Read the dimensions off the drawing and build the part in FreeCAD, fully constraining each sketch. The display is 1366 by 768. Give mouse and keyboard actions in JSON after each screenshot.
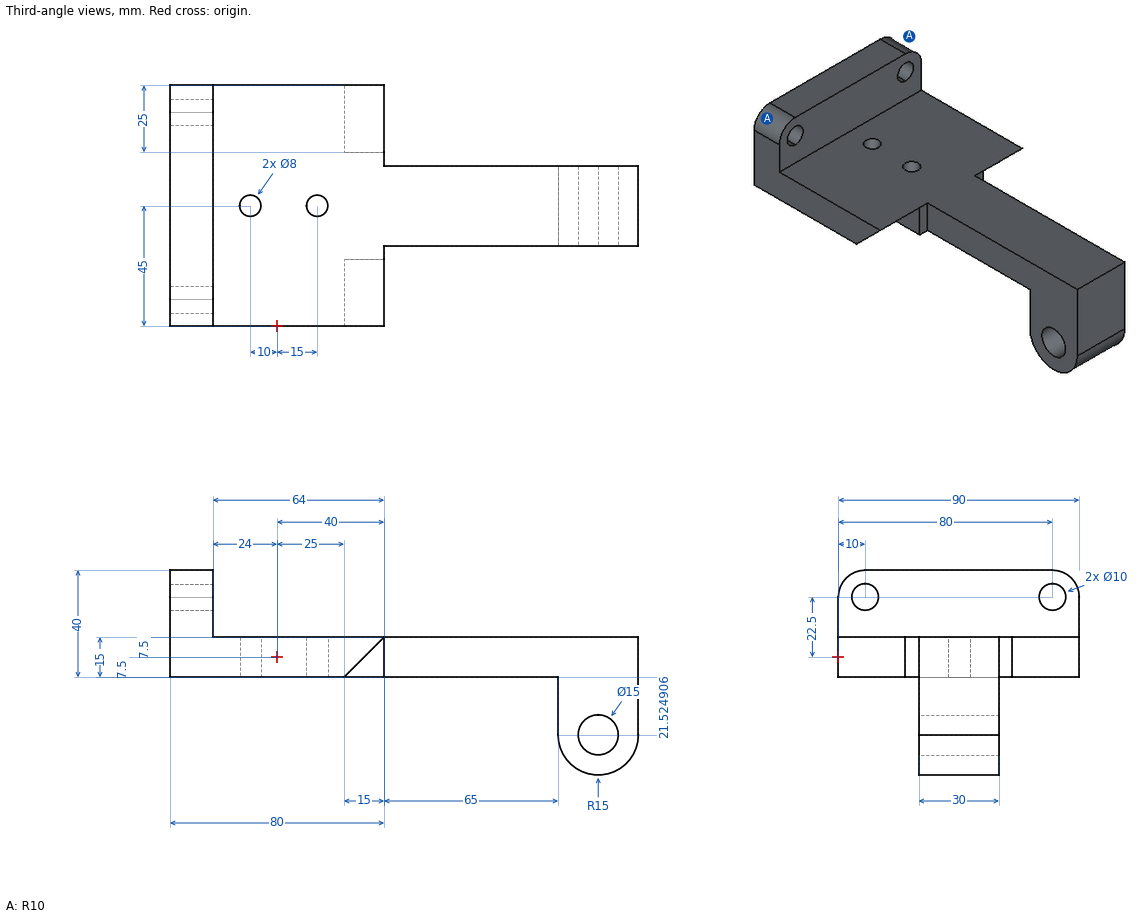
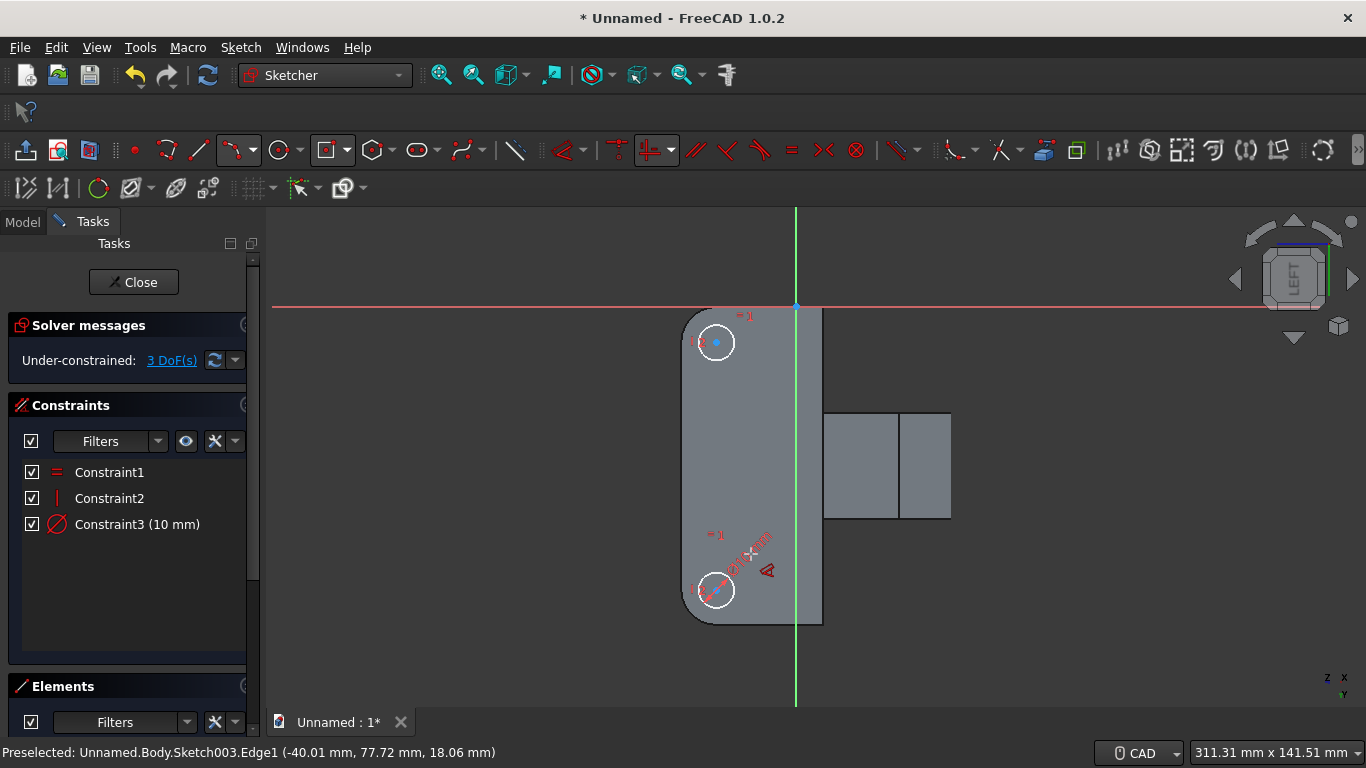
{"action": "left_click", "coordinate": [716, 590]}
{"action": "left_click", "coordinate": [830, 449]}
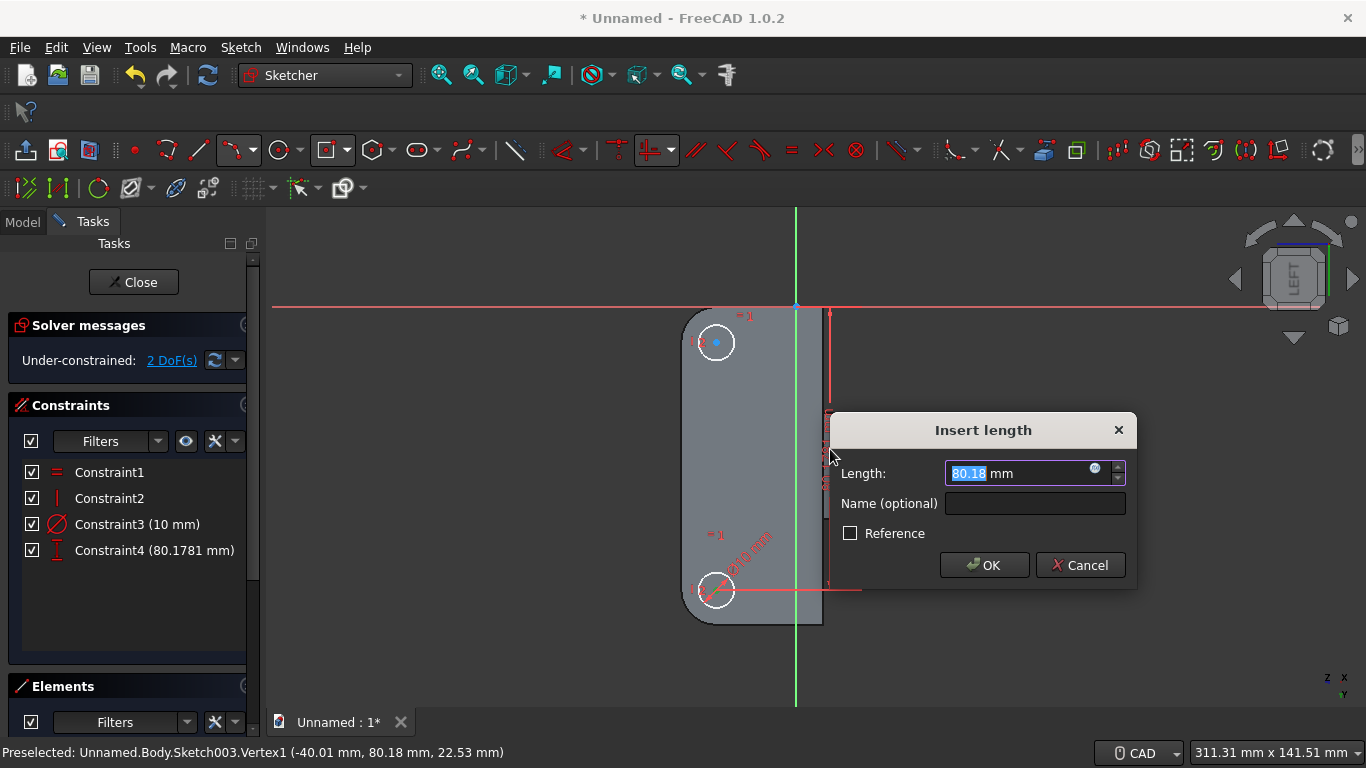
{"action": "type", "text": "80"}
{"action": "key", "text": "Return"}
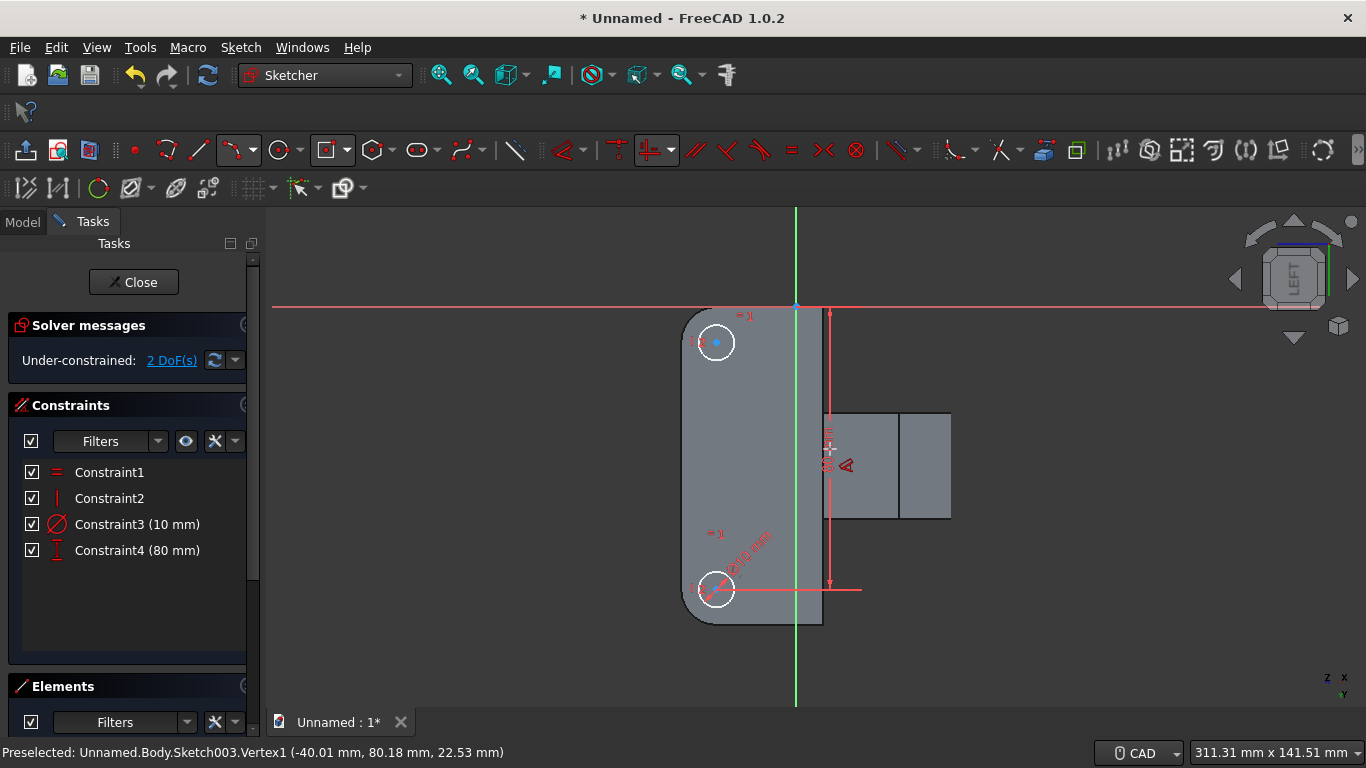
{"action": "left_click", "coordinate": [716, 343]}
{"action": "left_click", "coordinate": [830, 325]}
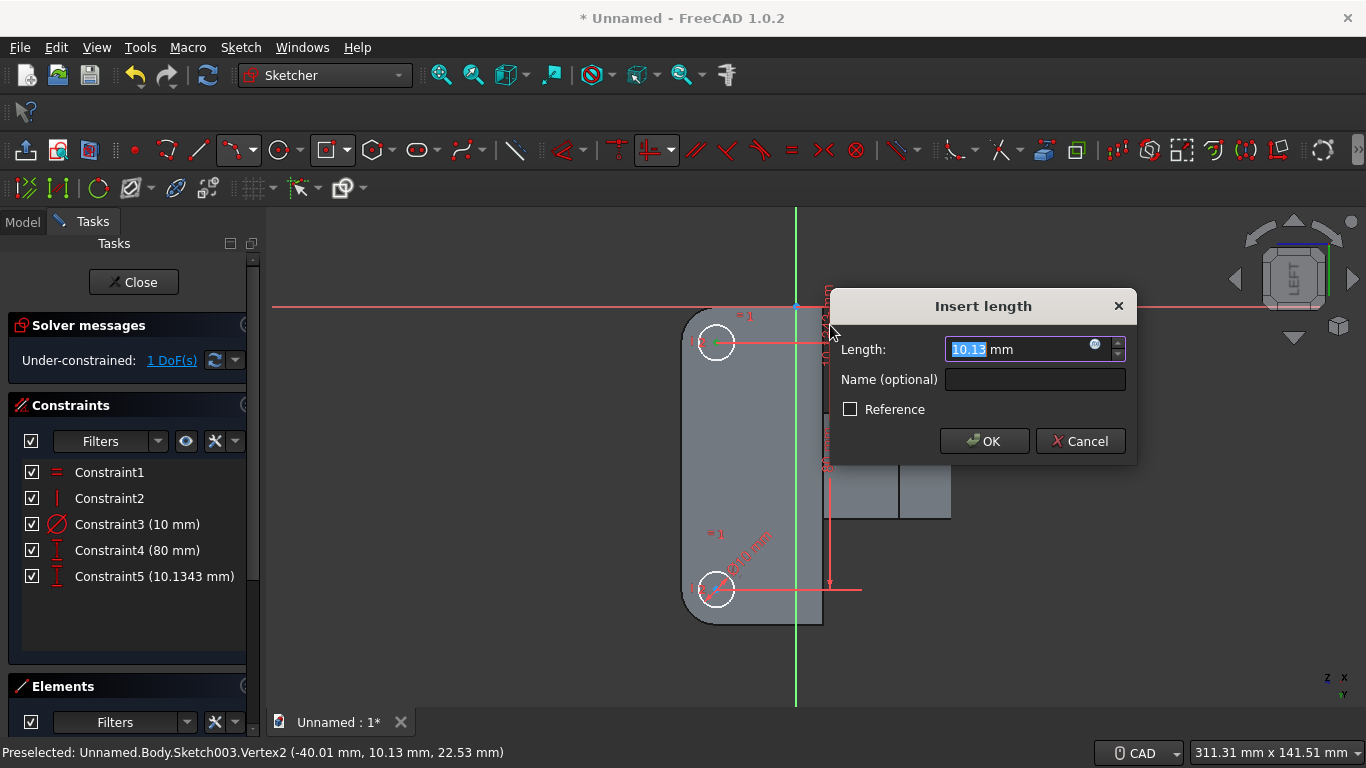
{"action": "type", "text": "10"}
{"action": "key", "text": "Return"}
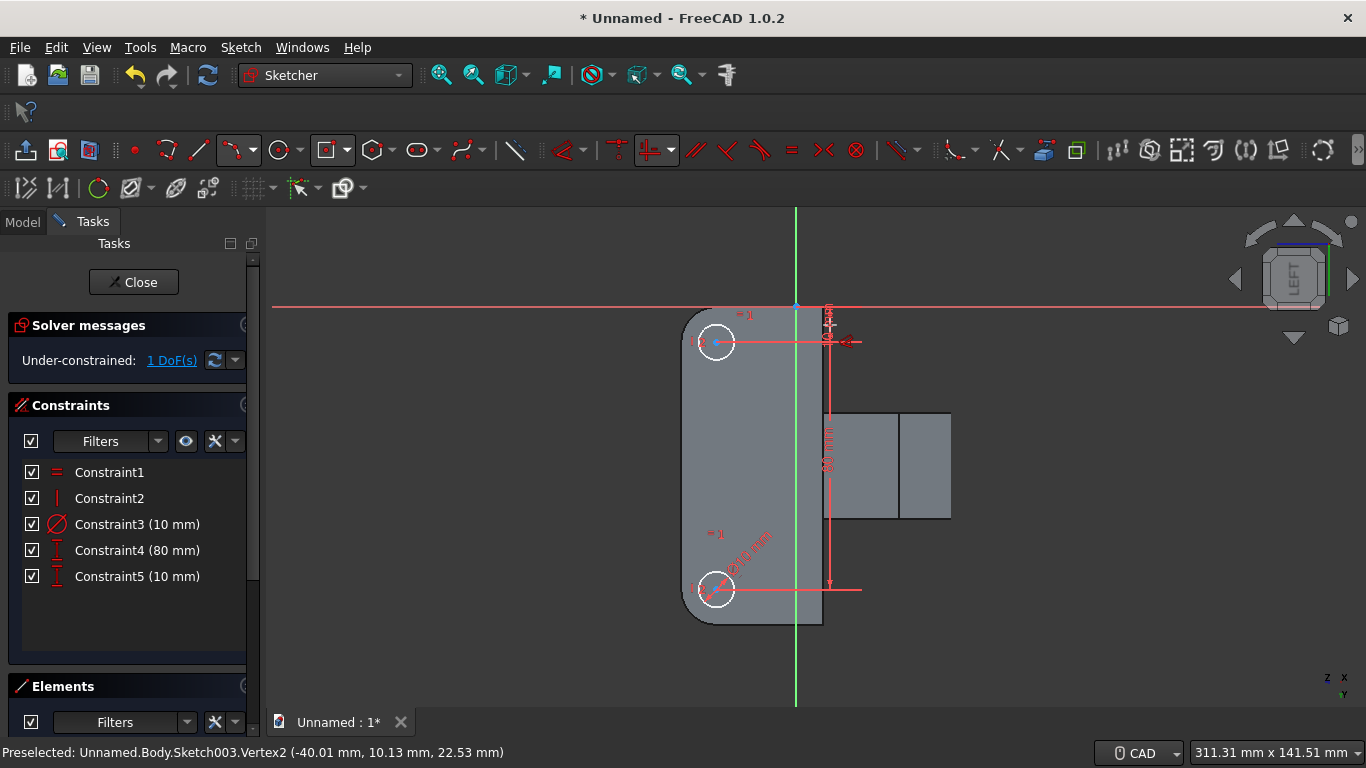
{"action": "left_click", "coordinate": [716, 590]}
{"action": "left_click", "coordinate": [756, 273]}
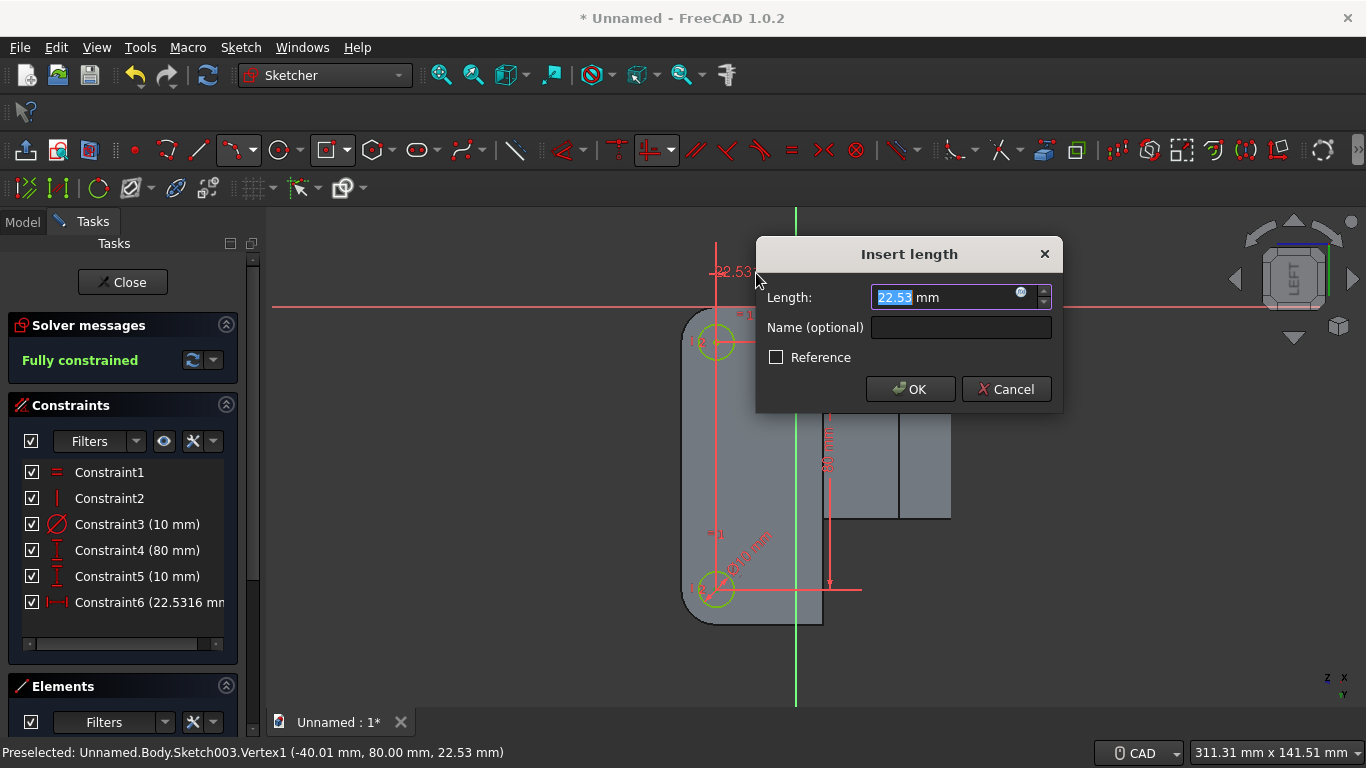
{"action": "type", "text": "22.5"}
{"action": "key", "text": "Return"}
{"action": "key", "text": "Escape"}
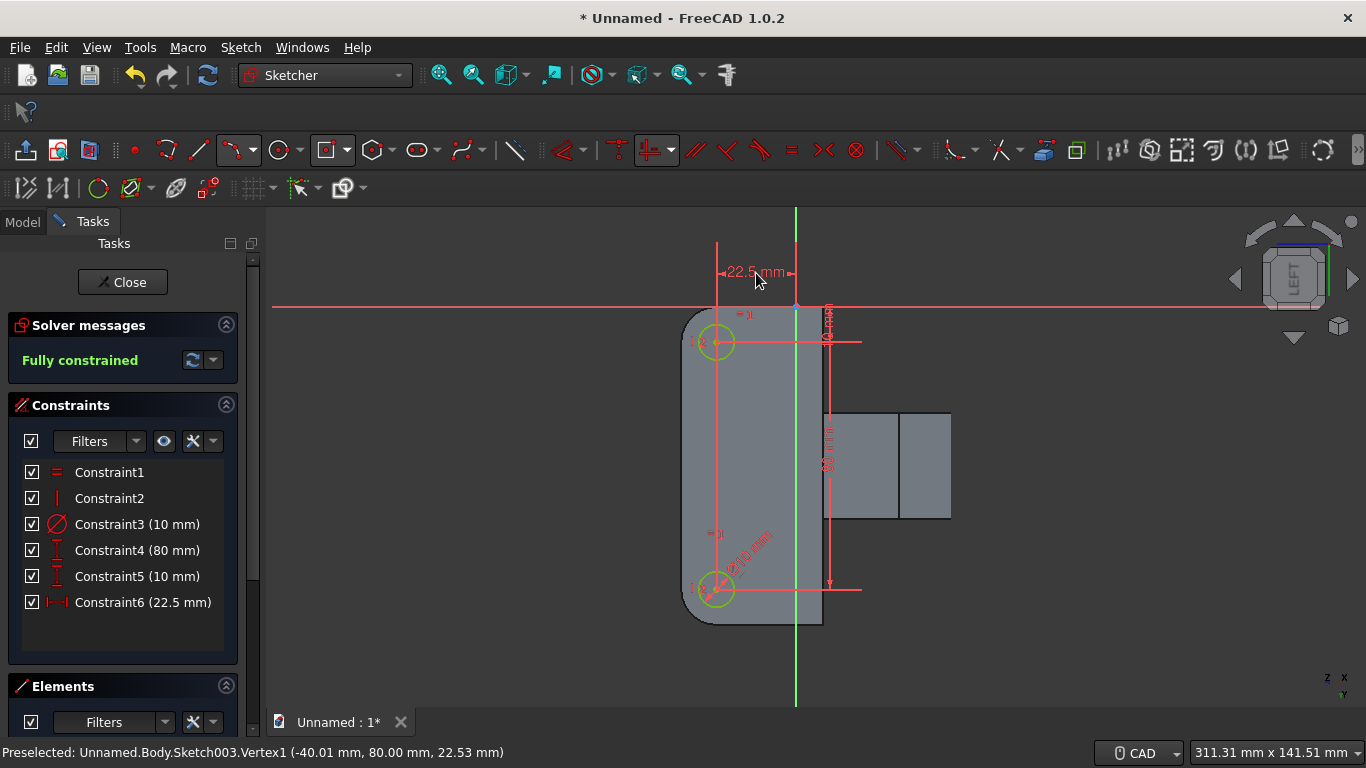
{"action": "left_click", "coordinate": [123, 282]}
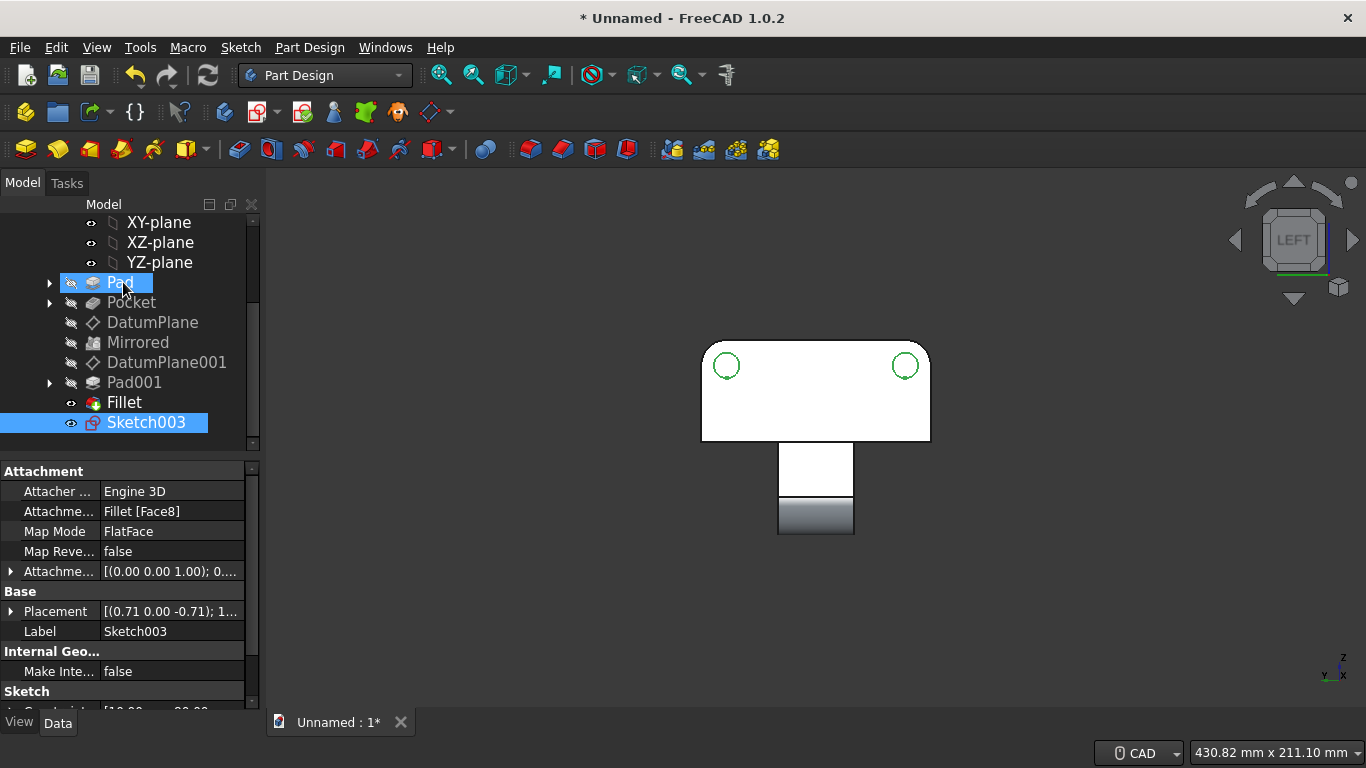
{"action": "left_click", "coordinate": [240, 150]}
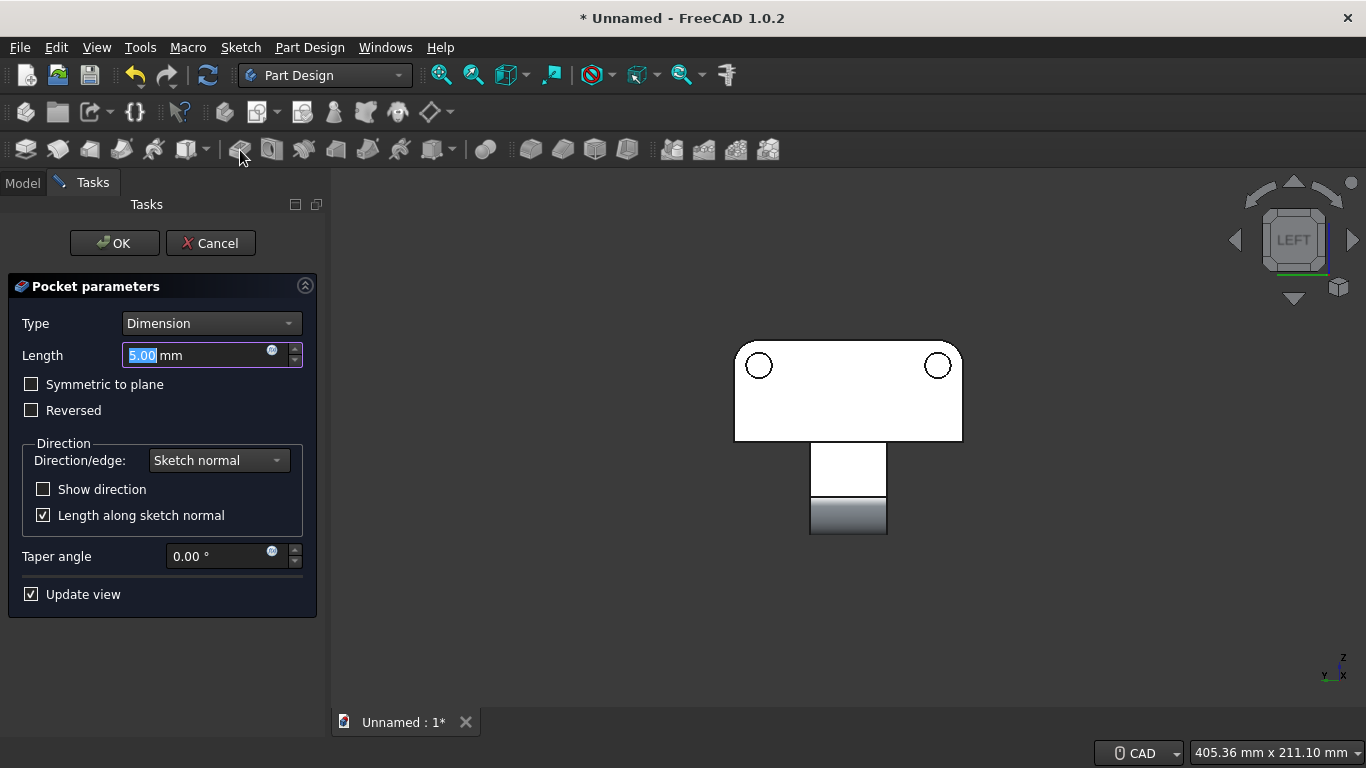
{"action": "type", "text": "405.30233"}
{"action": "key", "text": "Tab"}